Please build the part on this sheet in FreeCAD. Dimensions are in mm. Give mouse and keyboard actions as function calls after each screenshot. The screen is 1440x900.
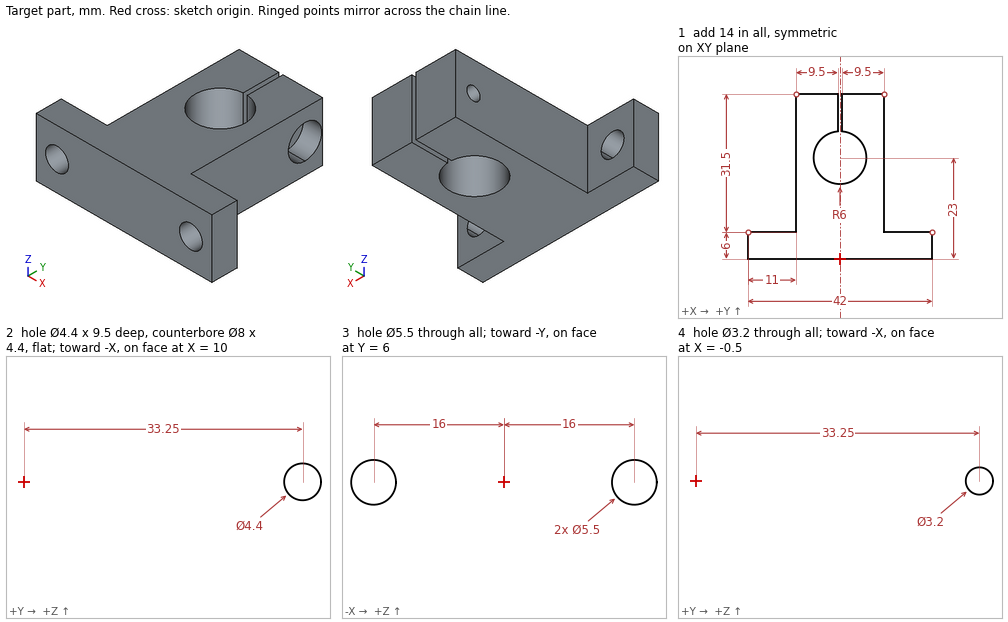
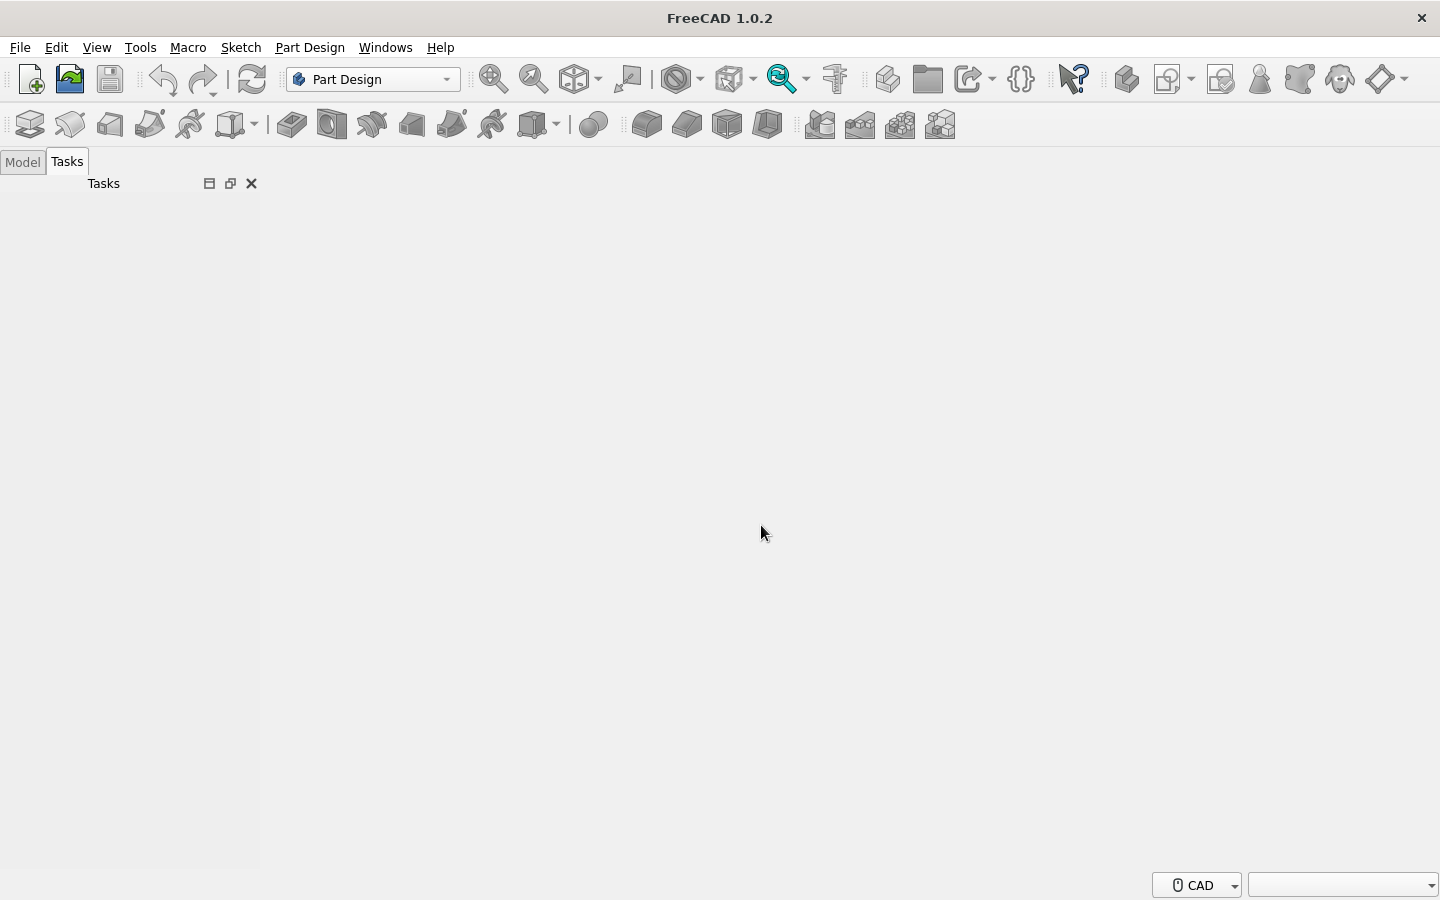
click(30, 80)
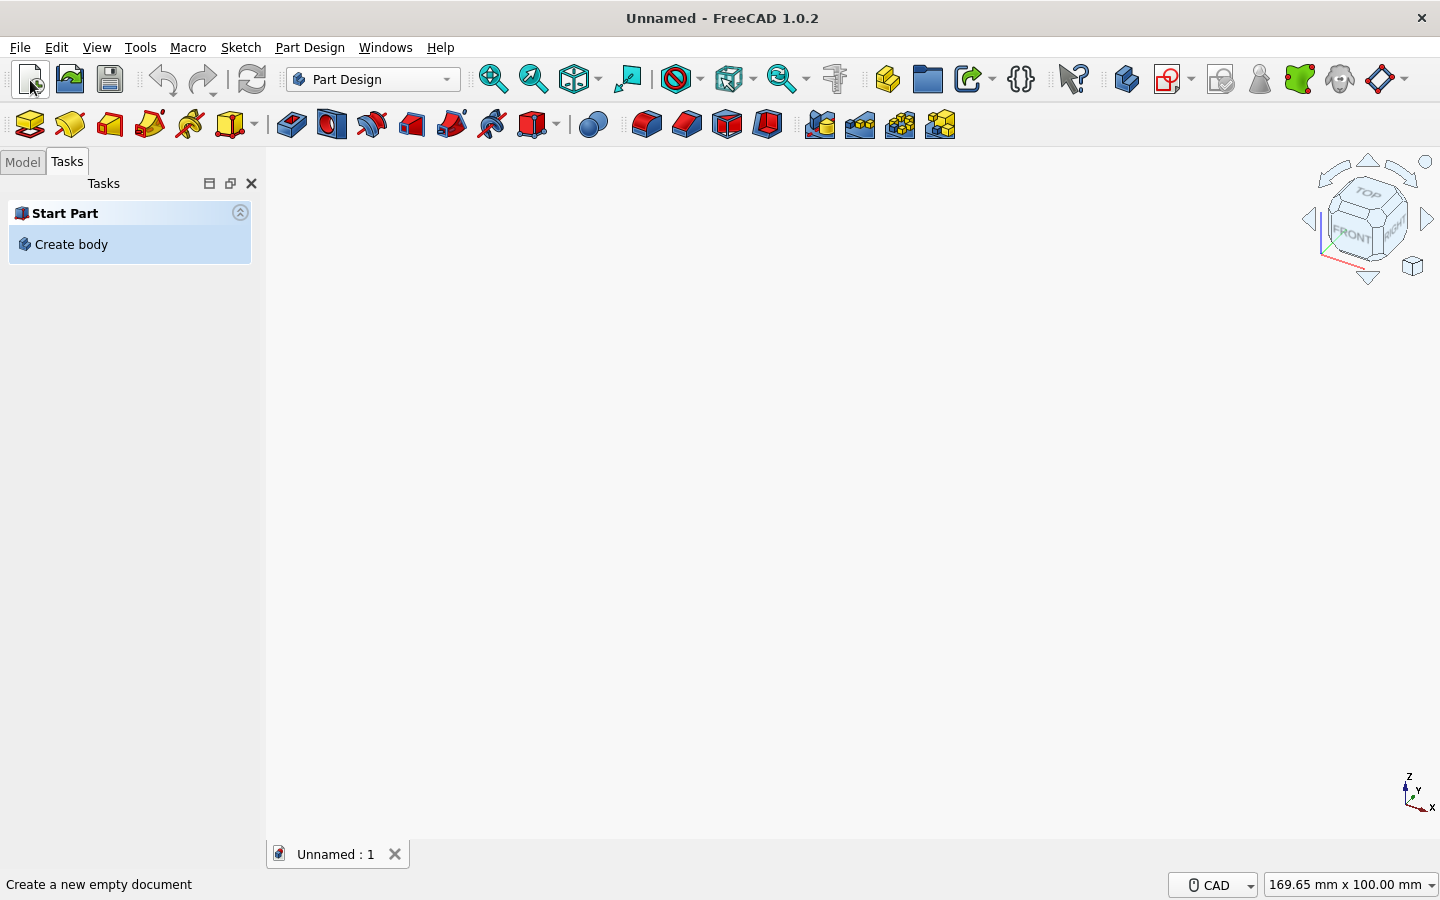
click(1168, 80)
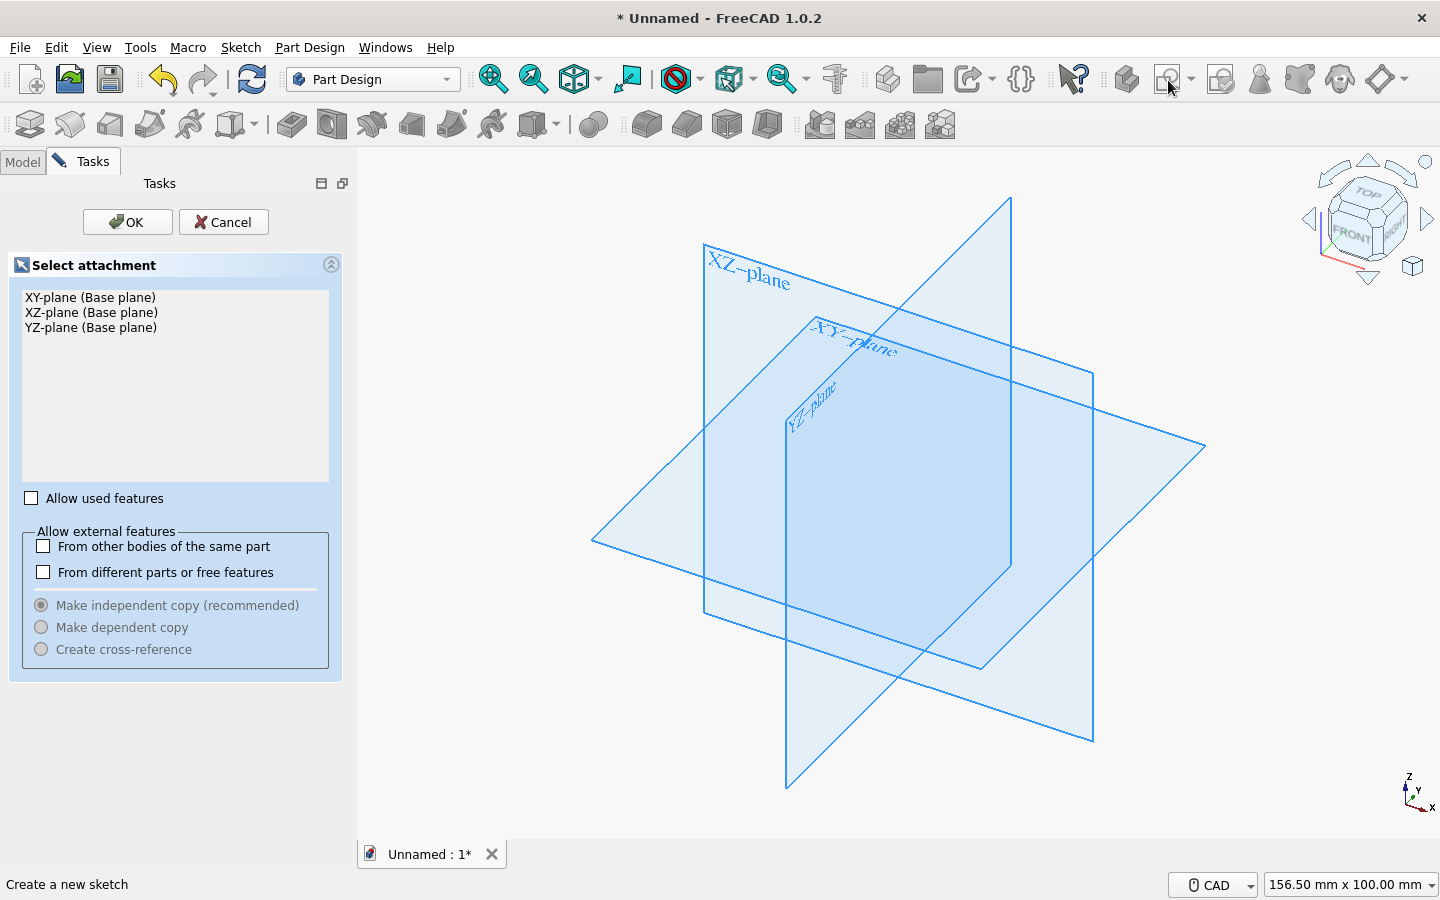
click(82, 298)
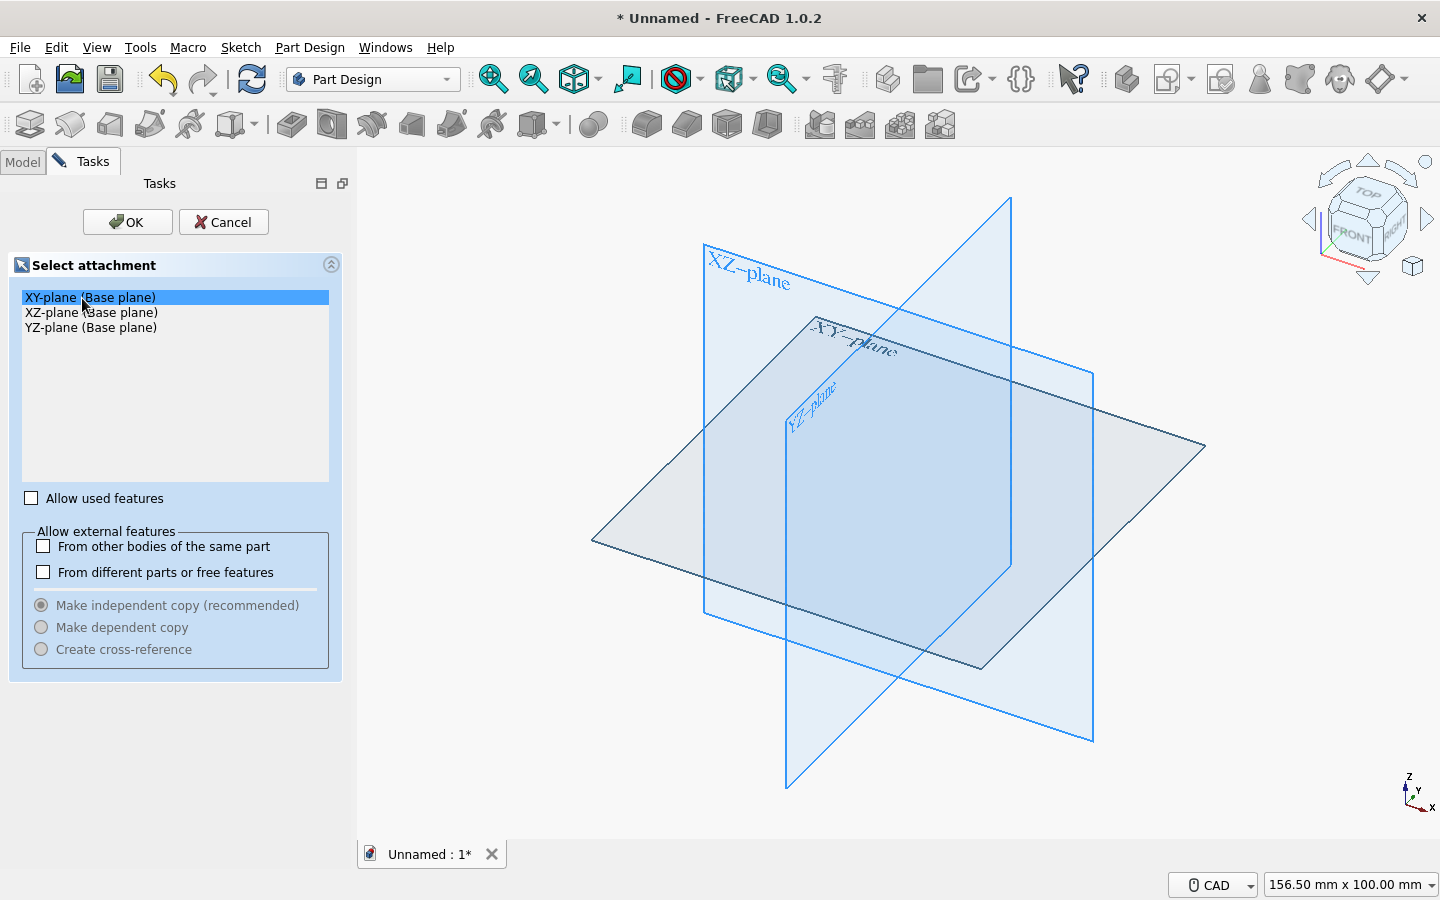
click(128, 222)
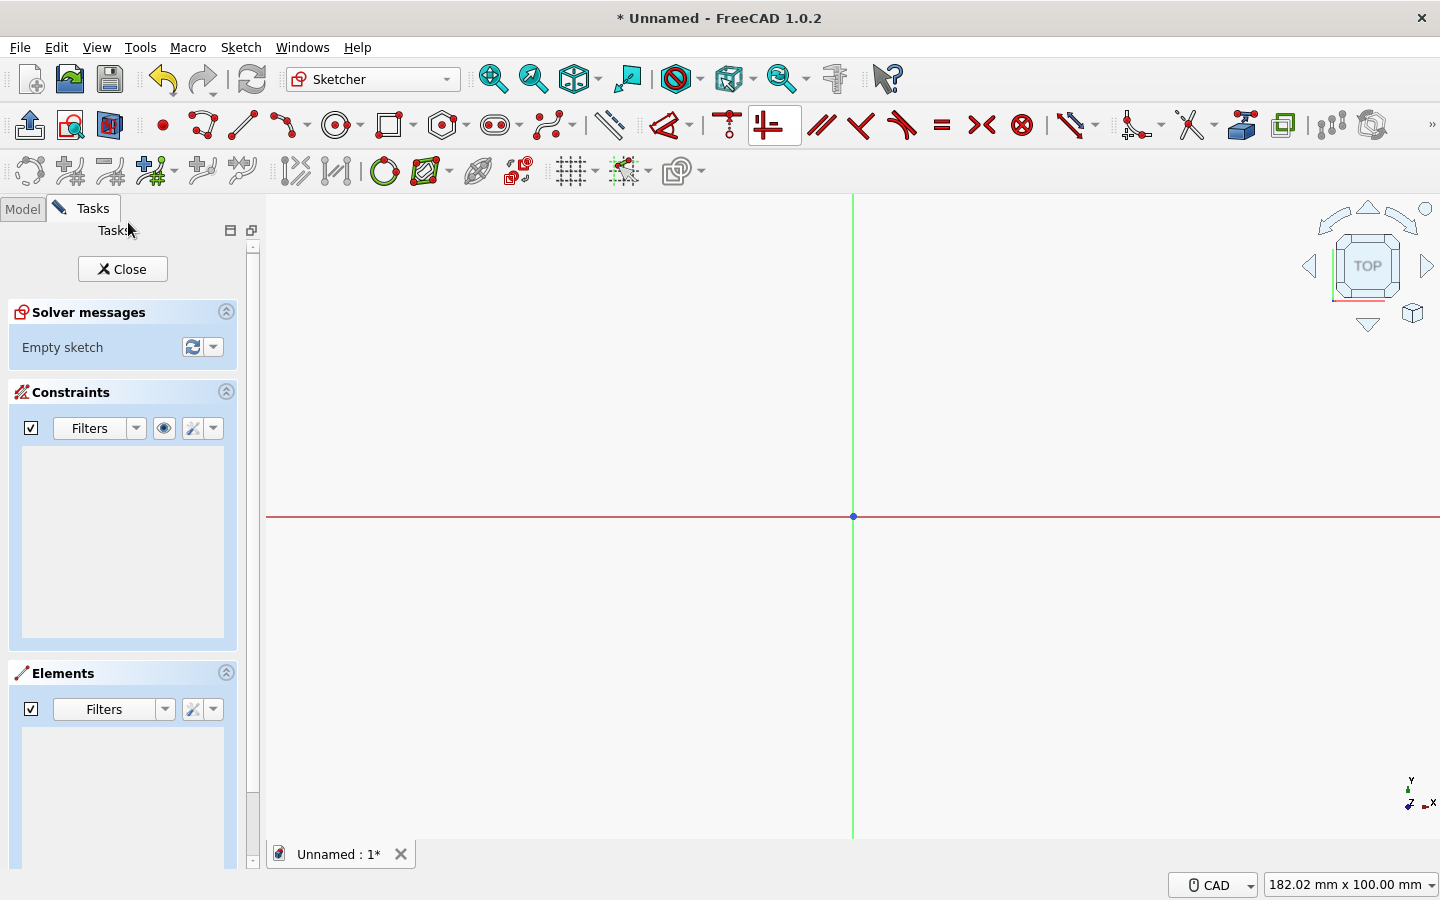
scroll(936, 248, up, 3)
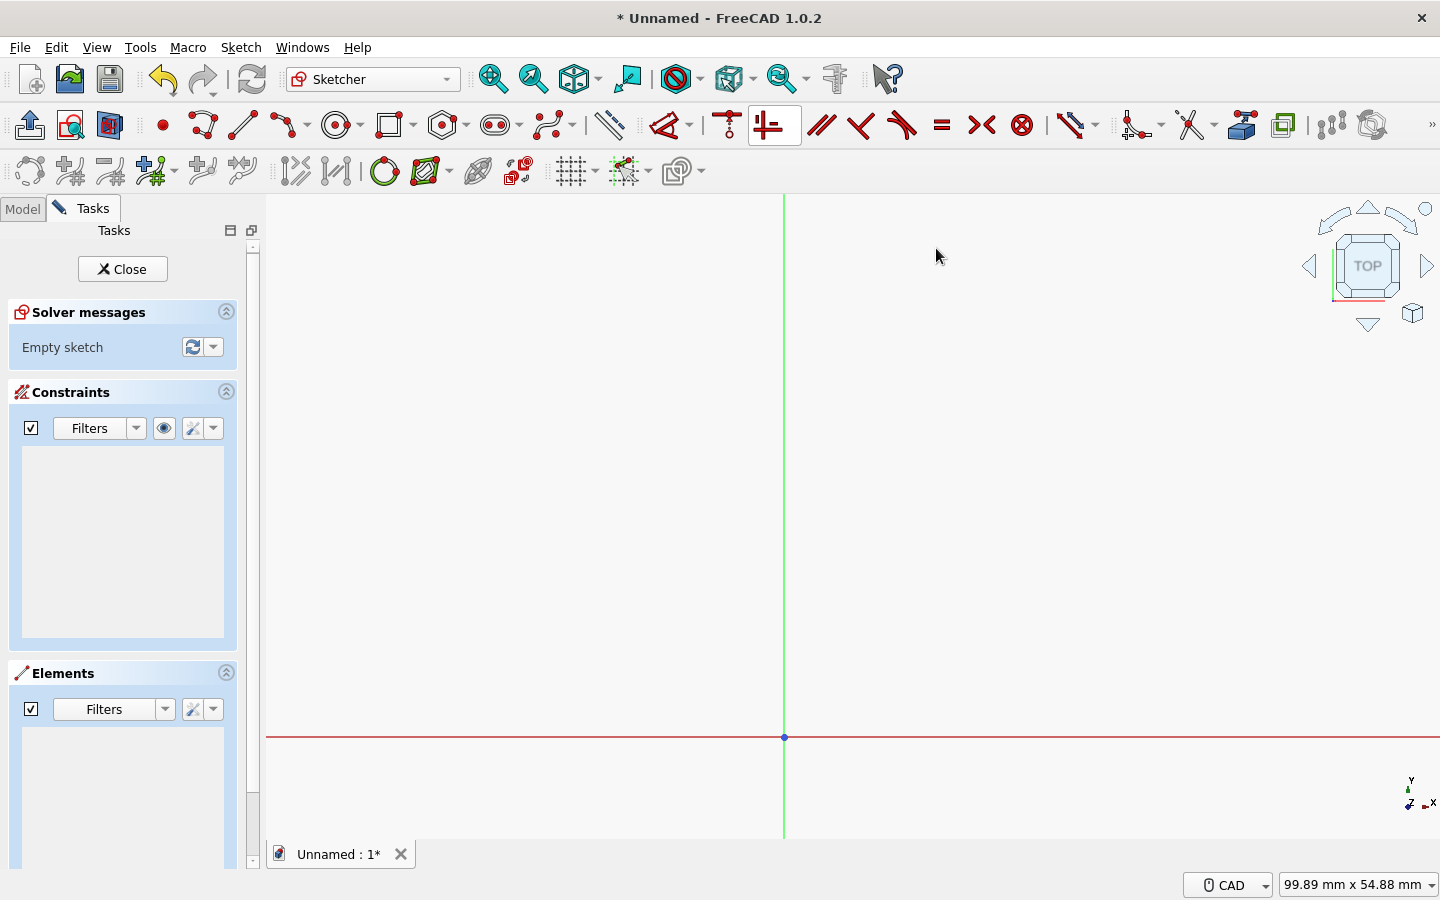
click(204, 126)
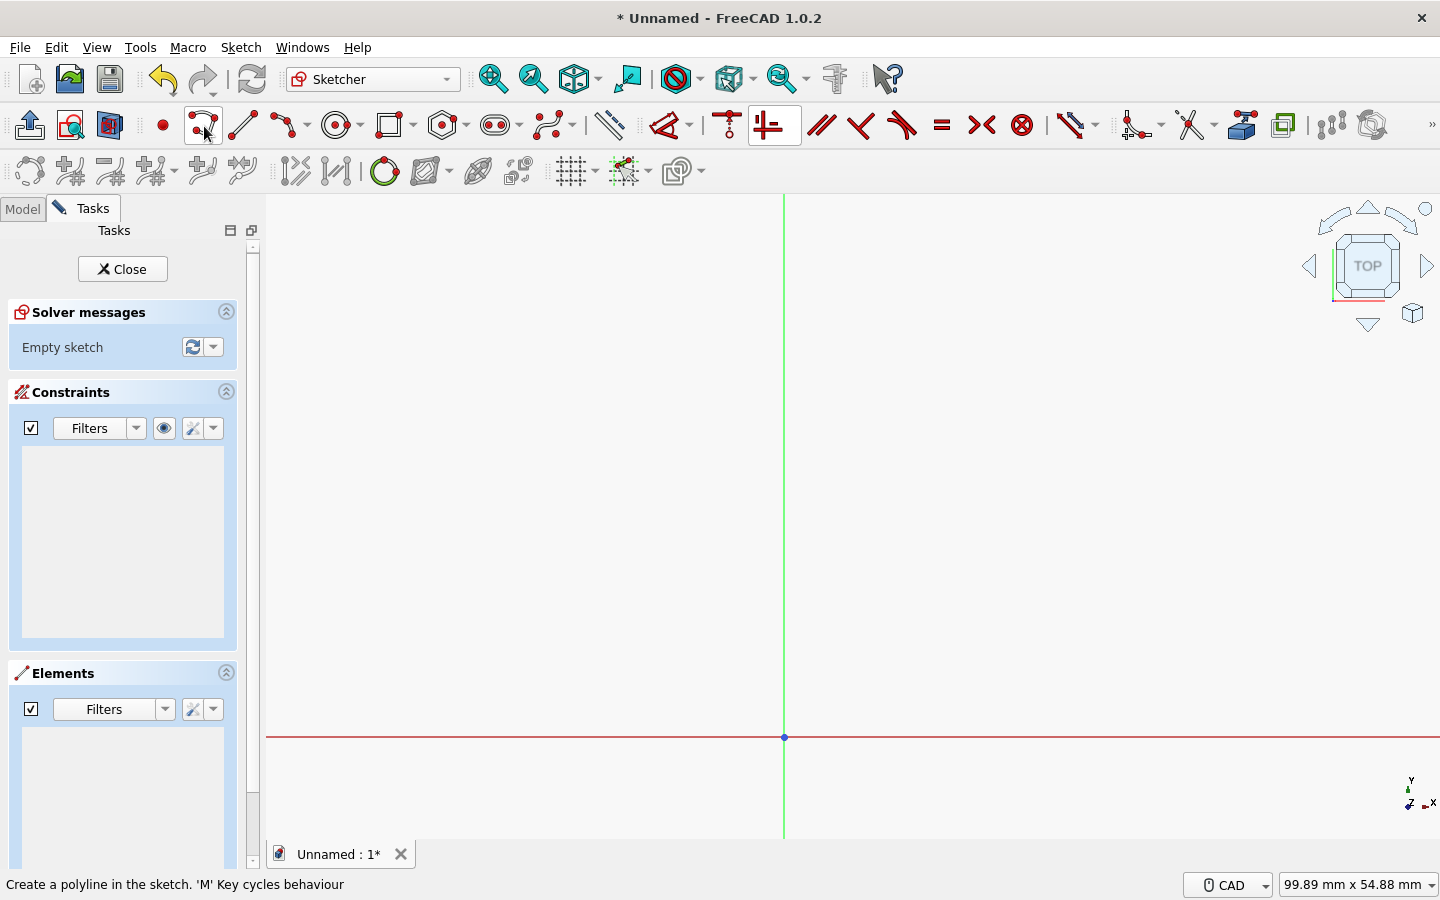
scroll(778, 397, up, 5)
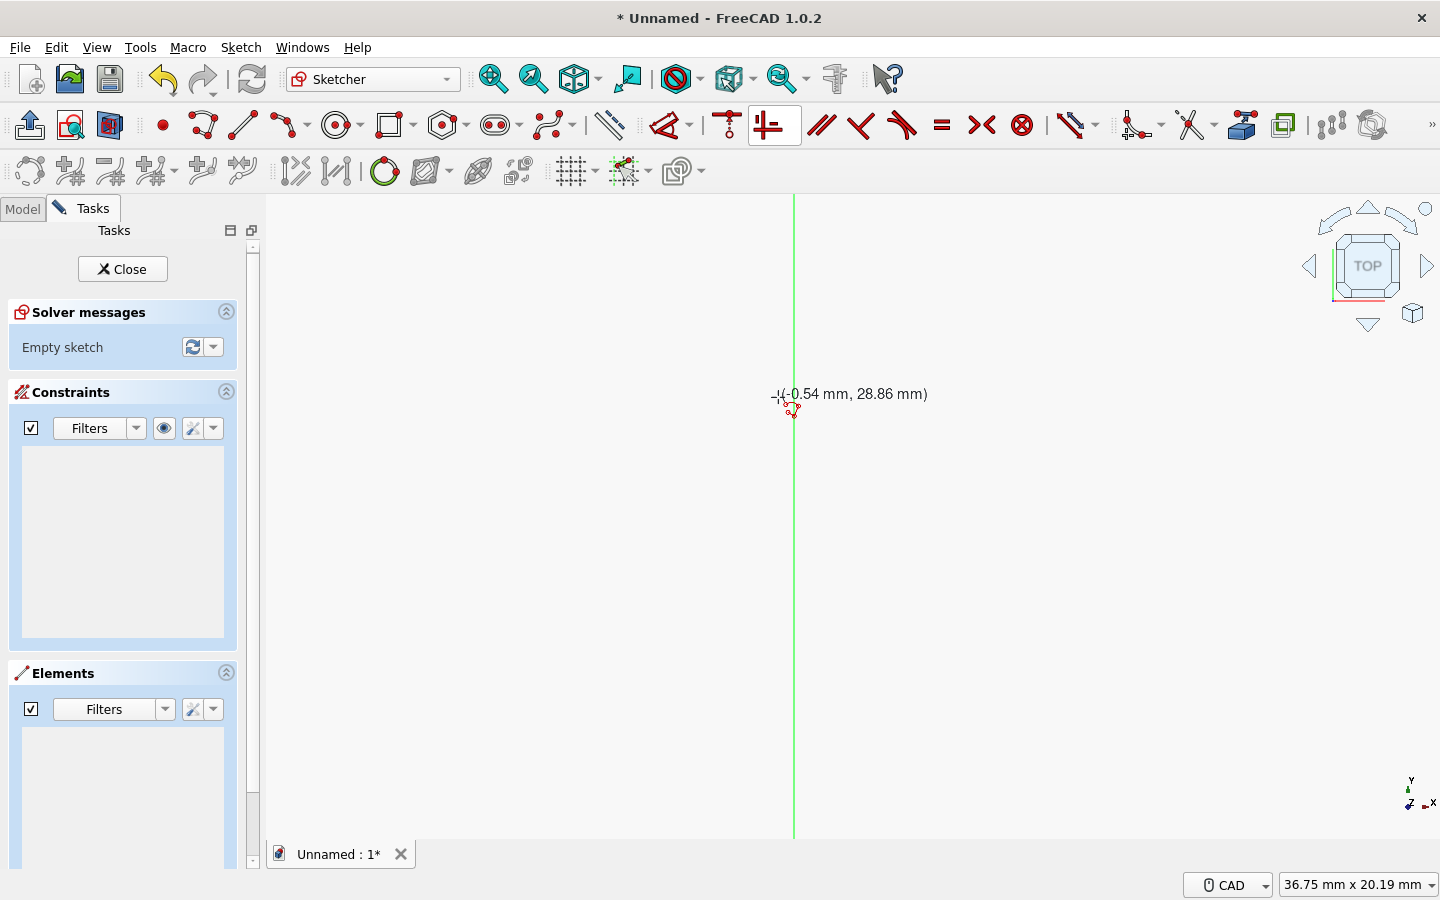
click(778, 395)